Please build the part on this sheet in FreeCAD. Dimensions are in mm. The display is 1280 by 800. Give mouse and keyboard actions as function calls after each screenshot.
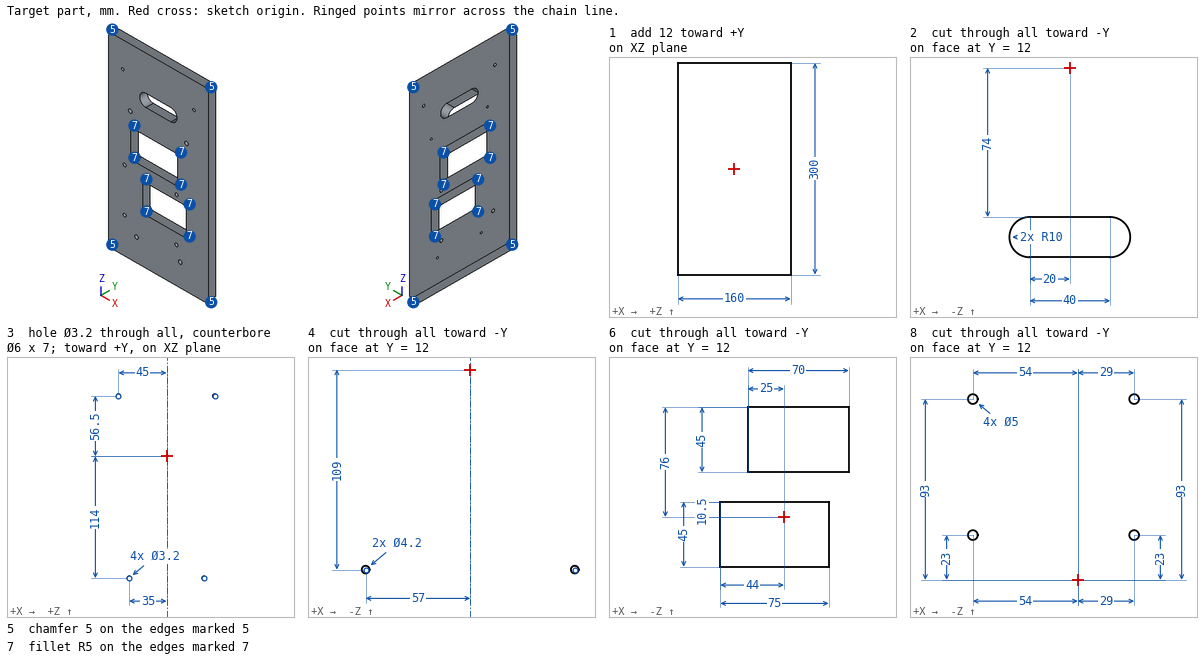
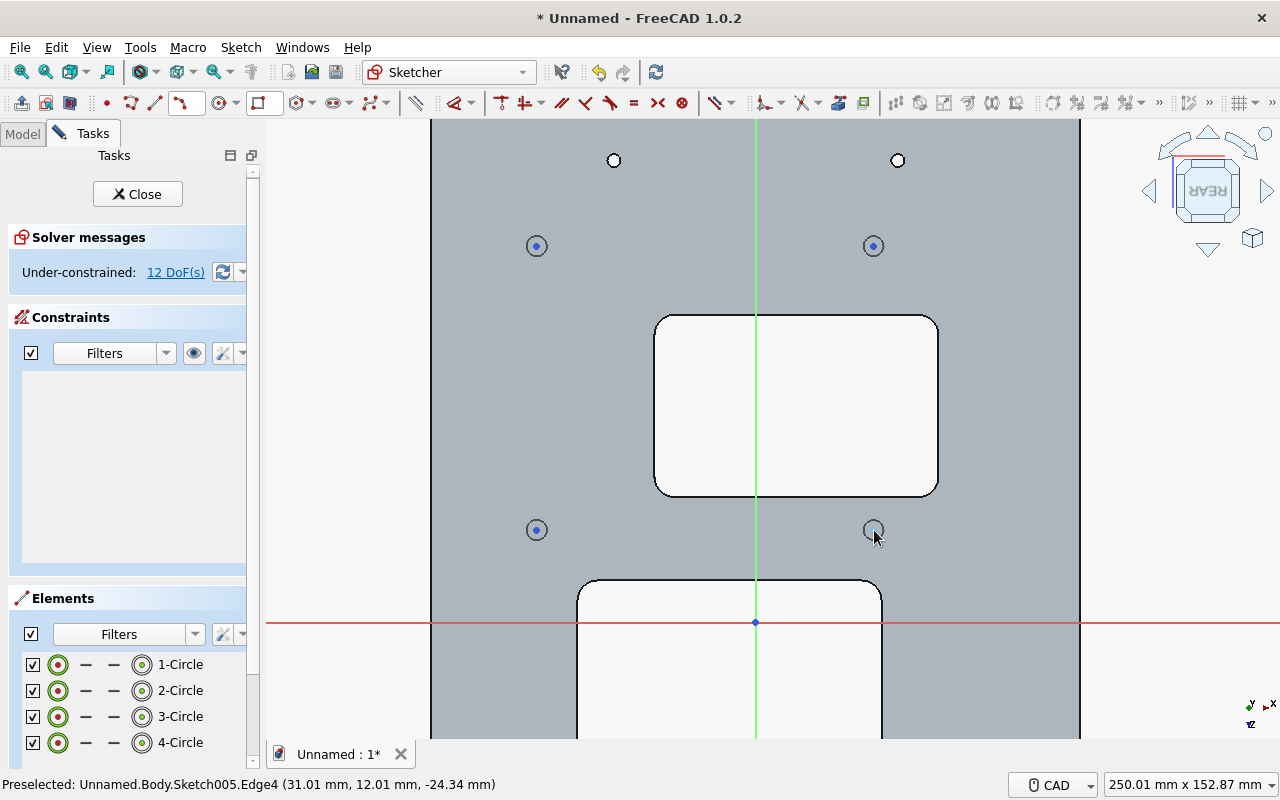
scroll(544, 239, up, 2)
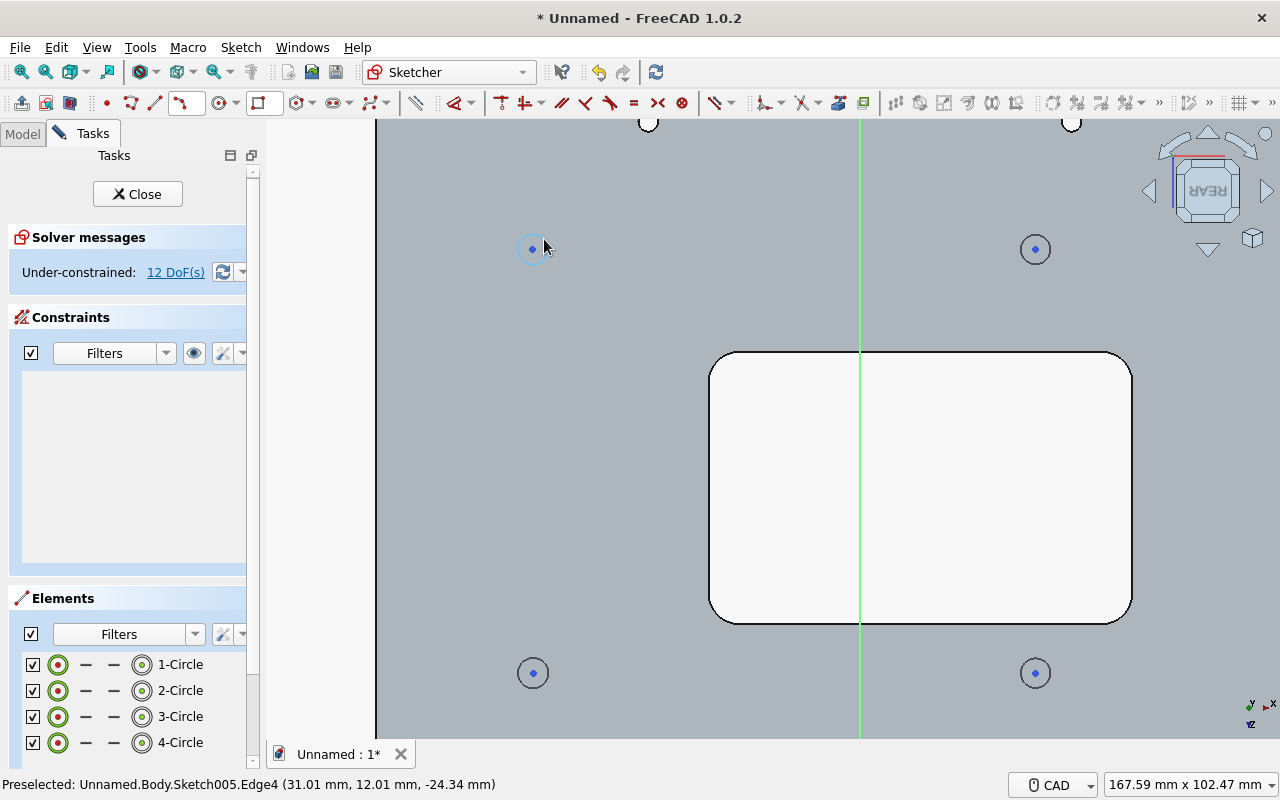
click(544, 239)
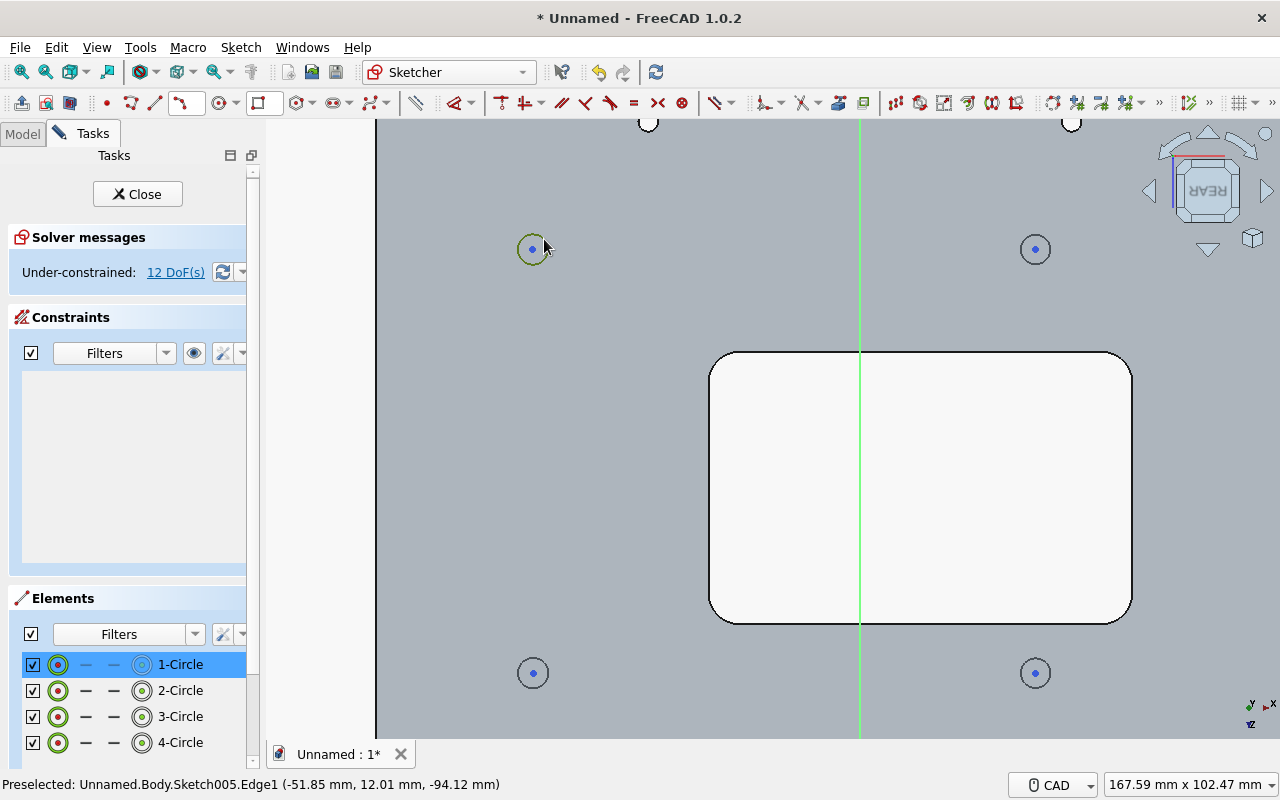
click(1046, 239)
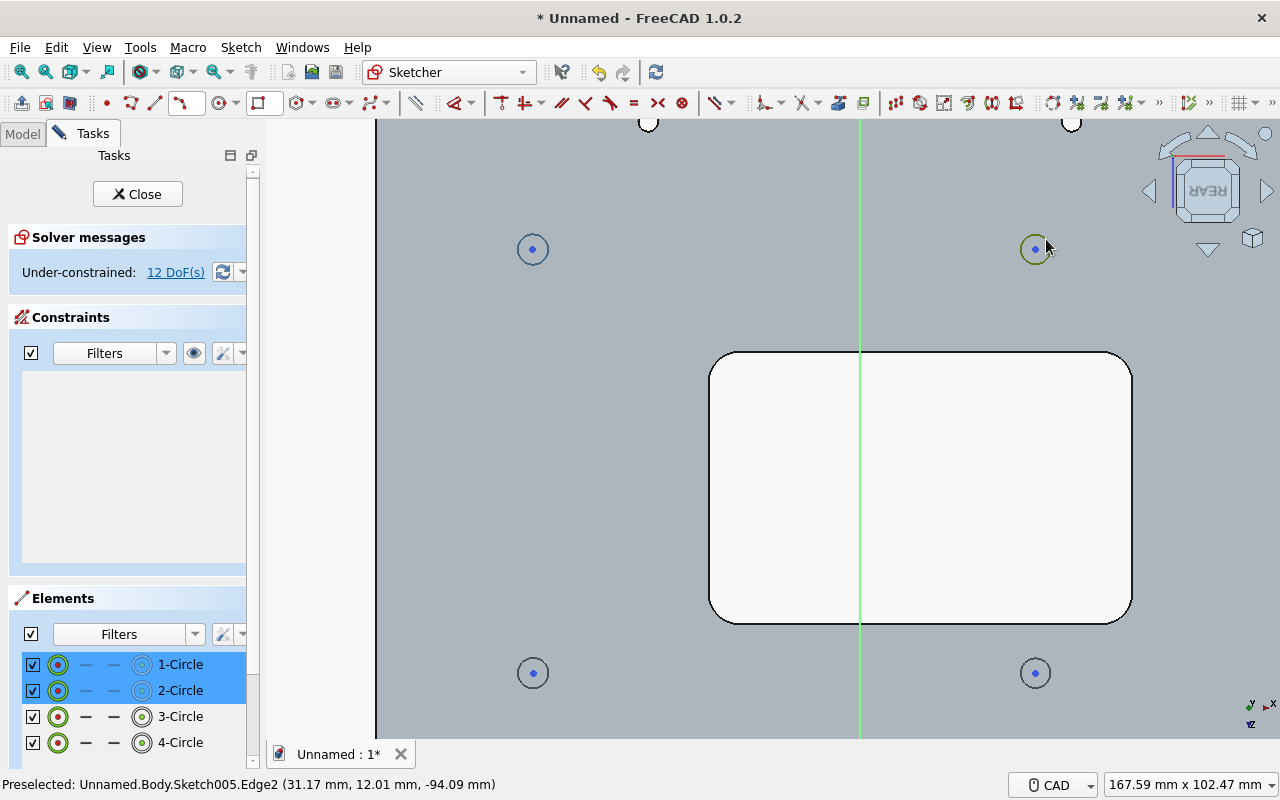
click(544, 662)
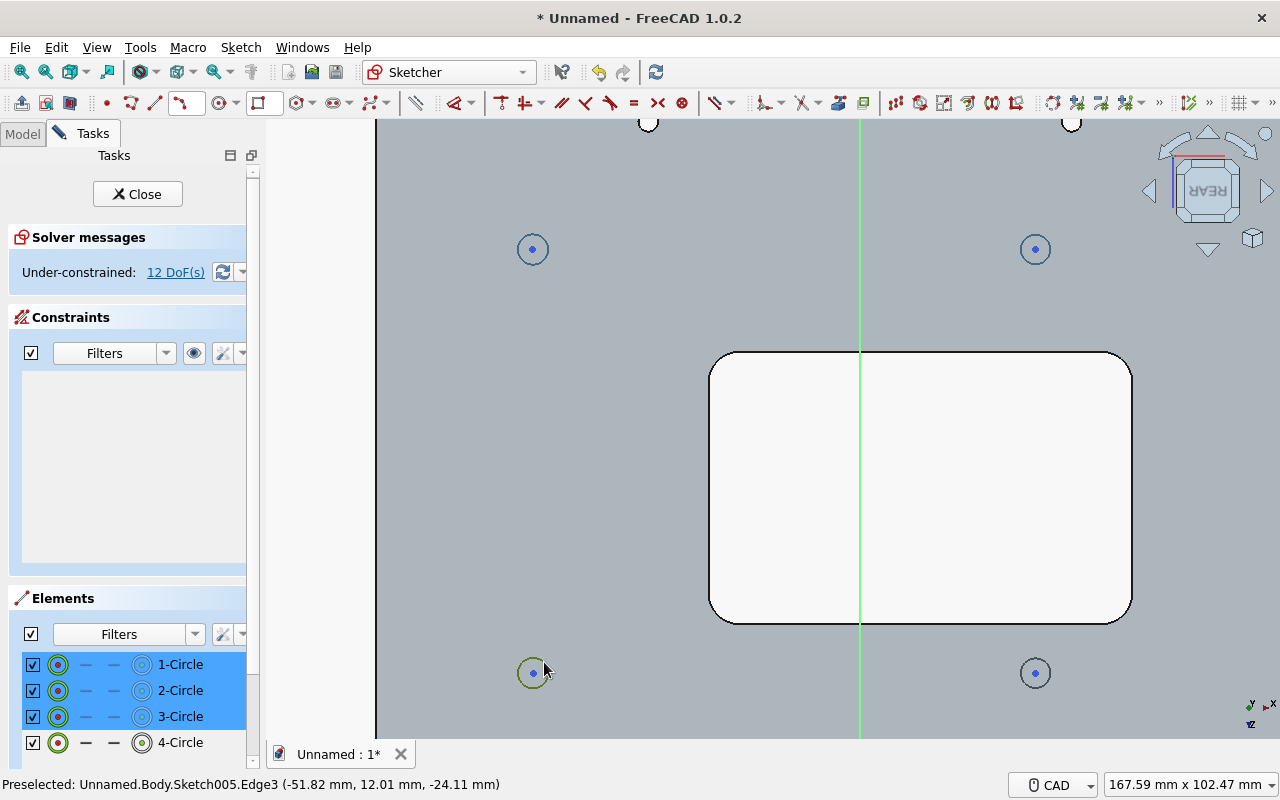
click(1046, 663)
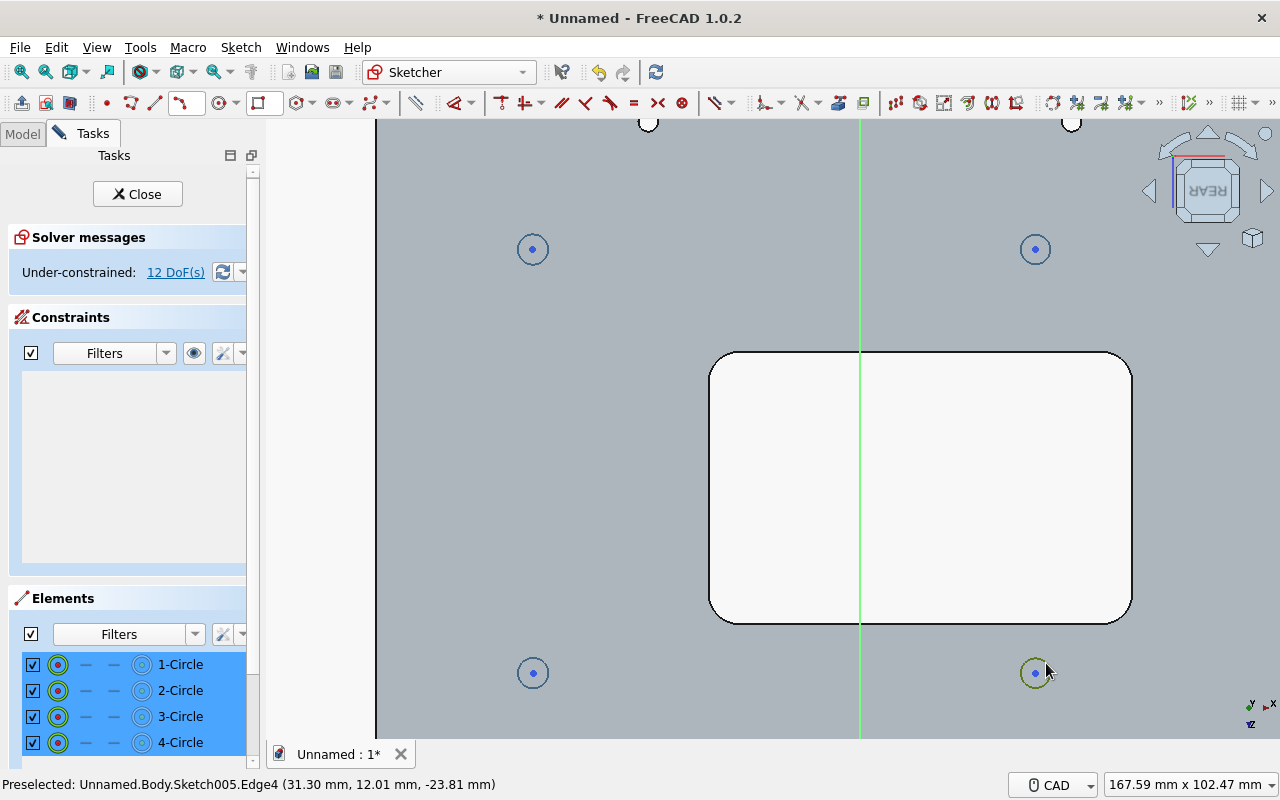
click(634, 104)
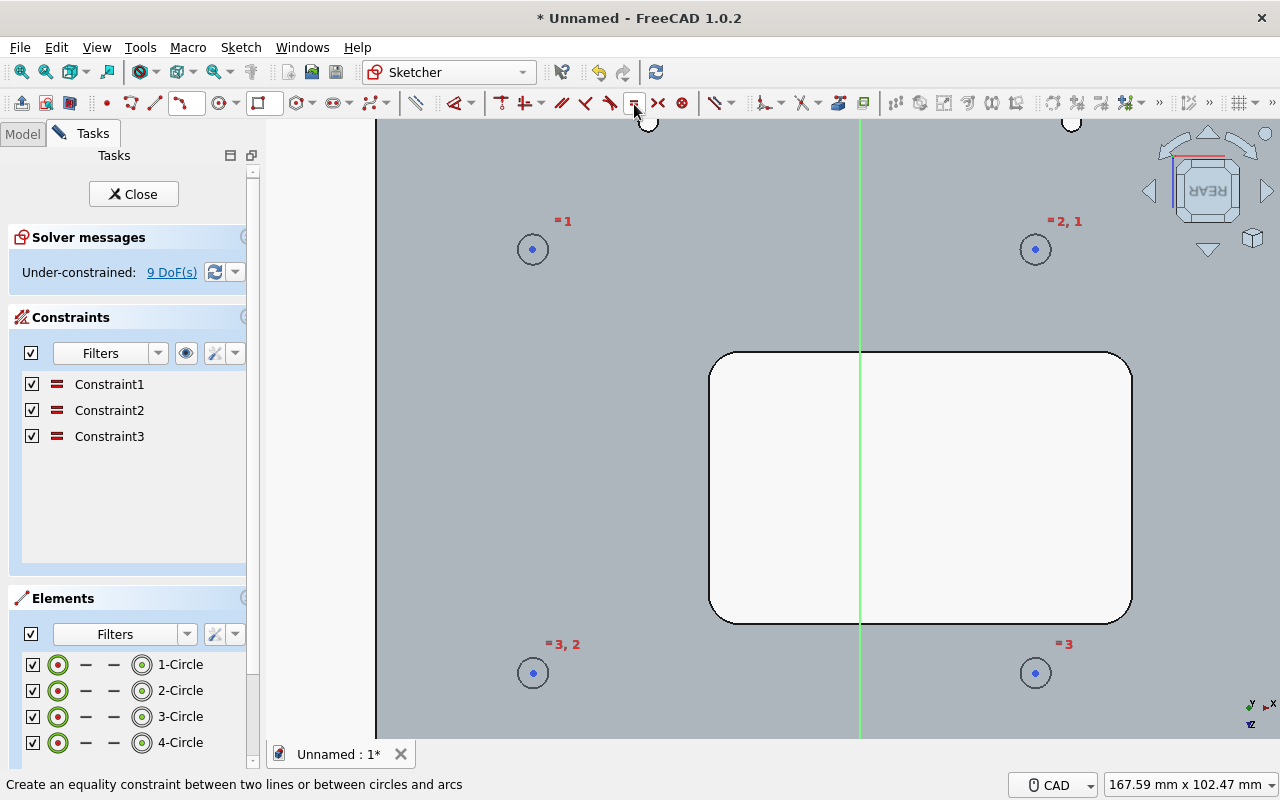
click(454, 104)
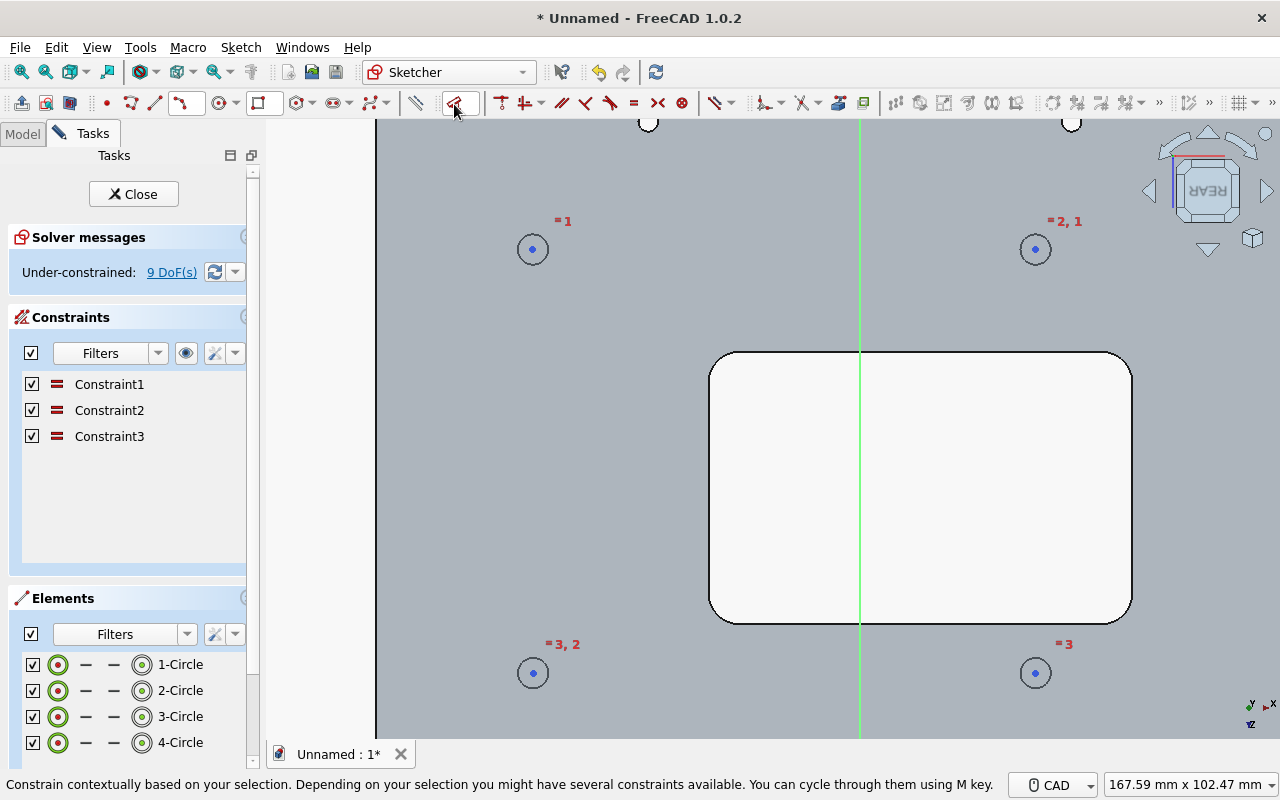
scroll(544, 239, up, 2)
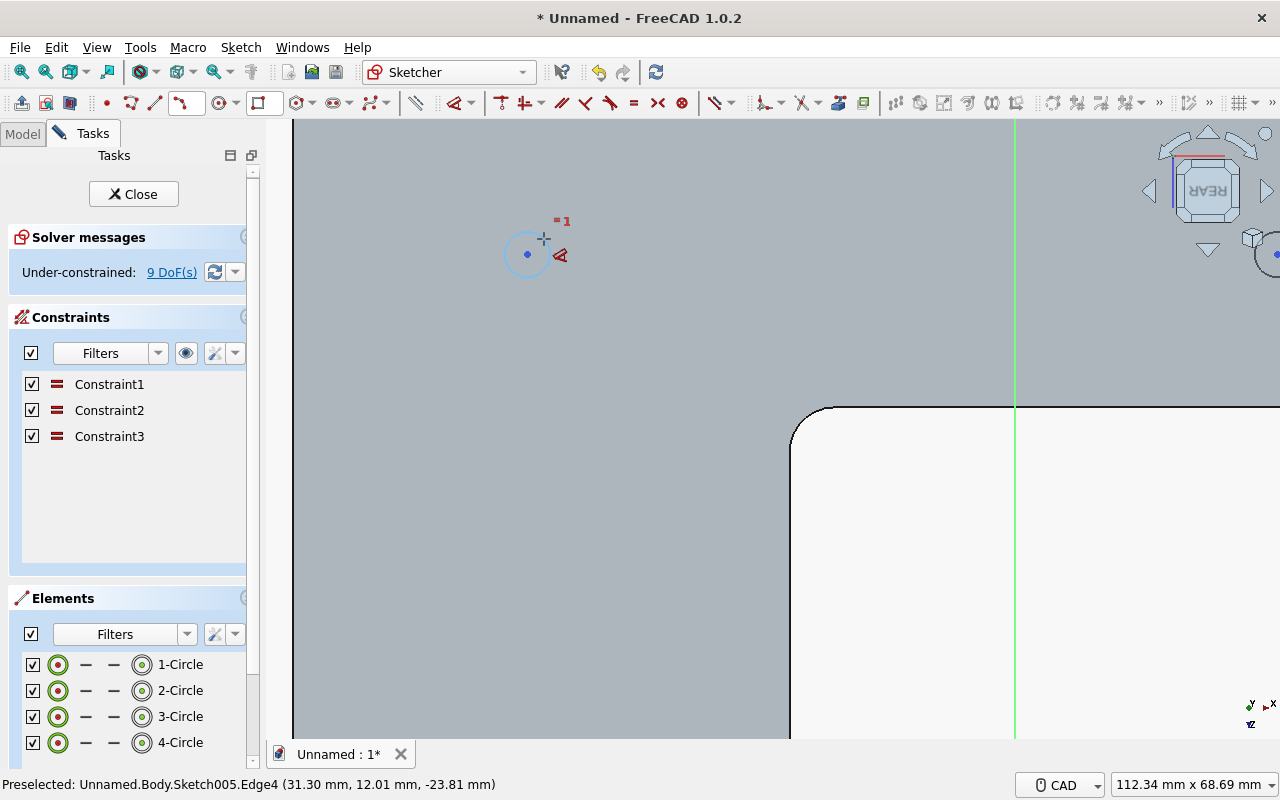
click(543, 239)
click(566, 216)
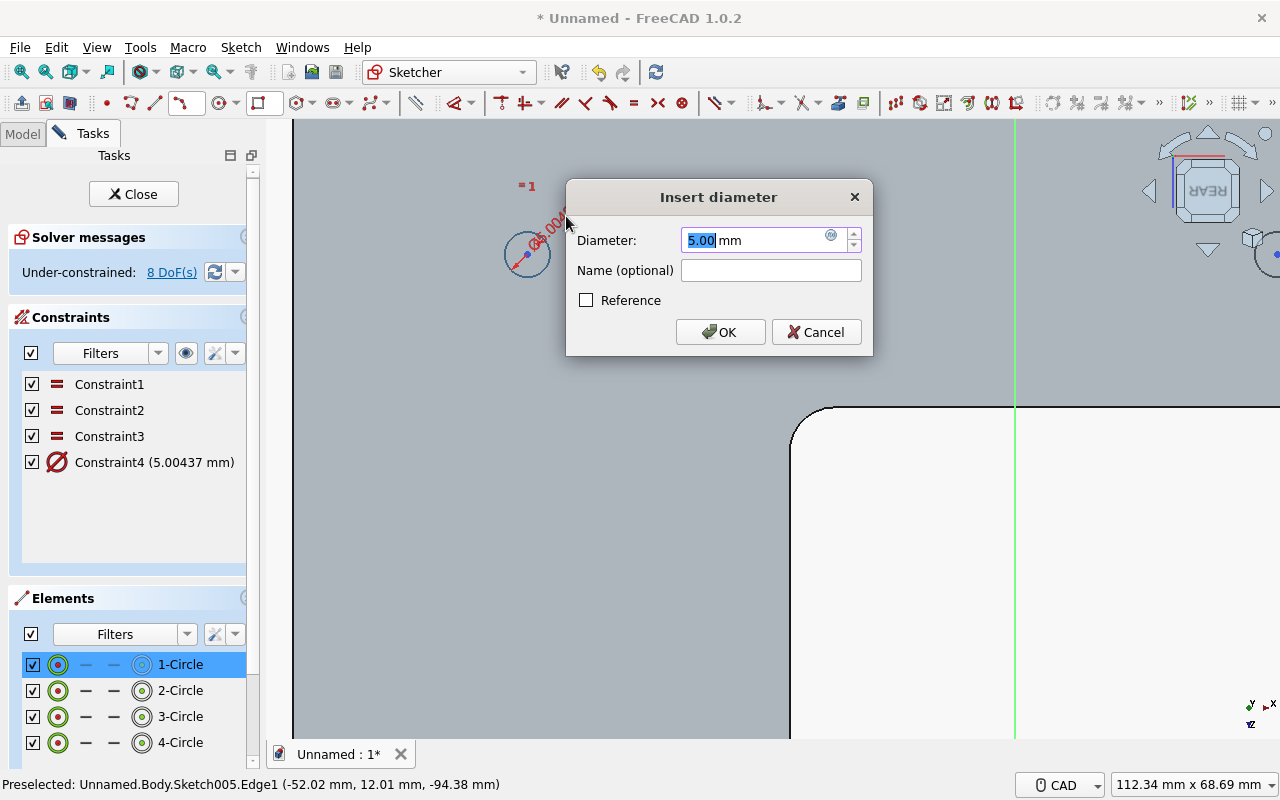
text(5)
key(Return)